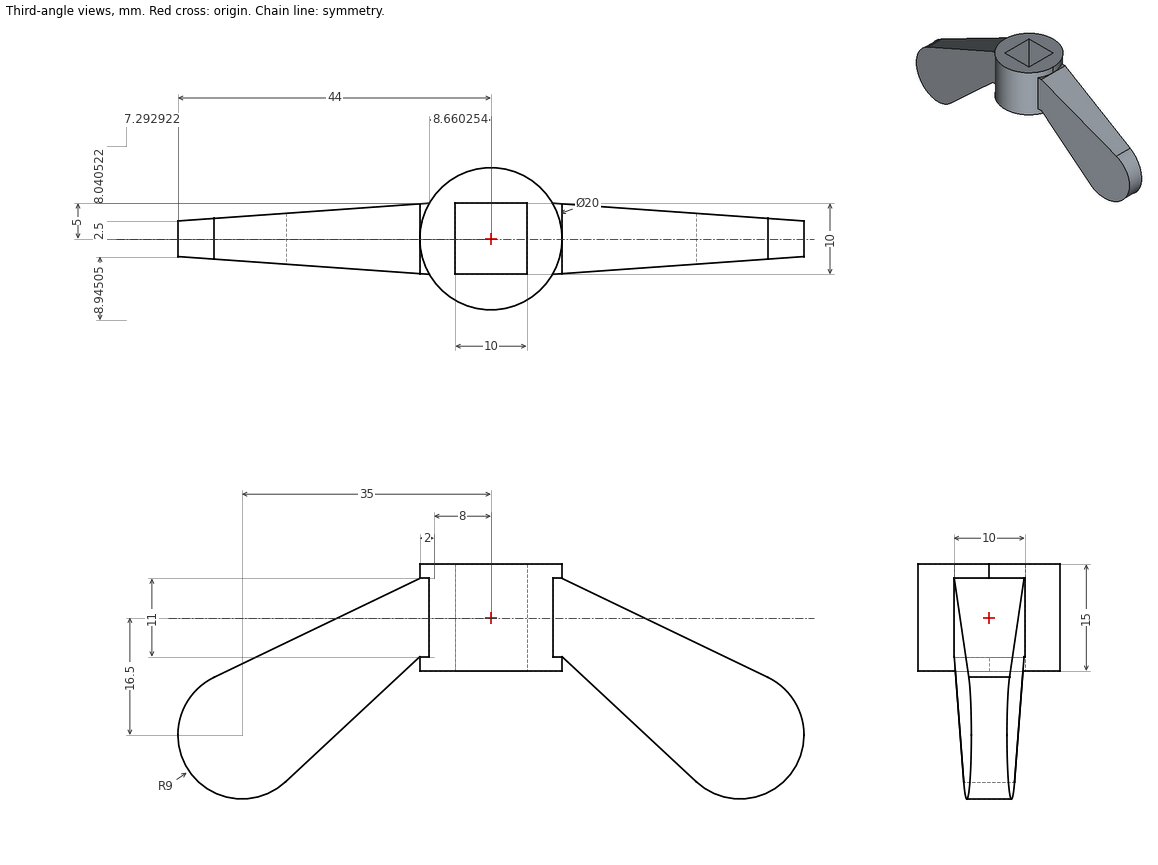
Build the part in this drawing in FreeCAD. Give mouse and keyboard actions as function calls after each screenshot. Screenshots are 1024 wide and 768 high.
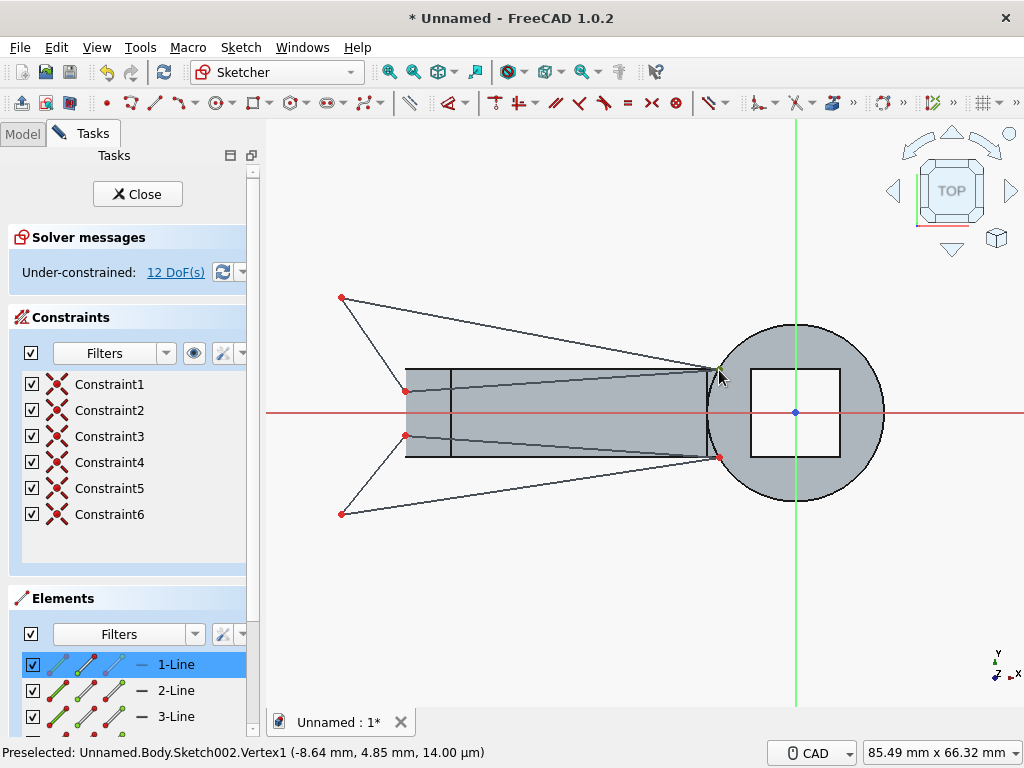
click(719, 458)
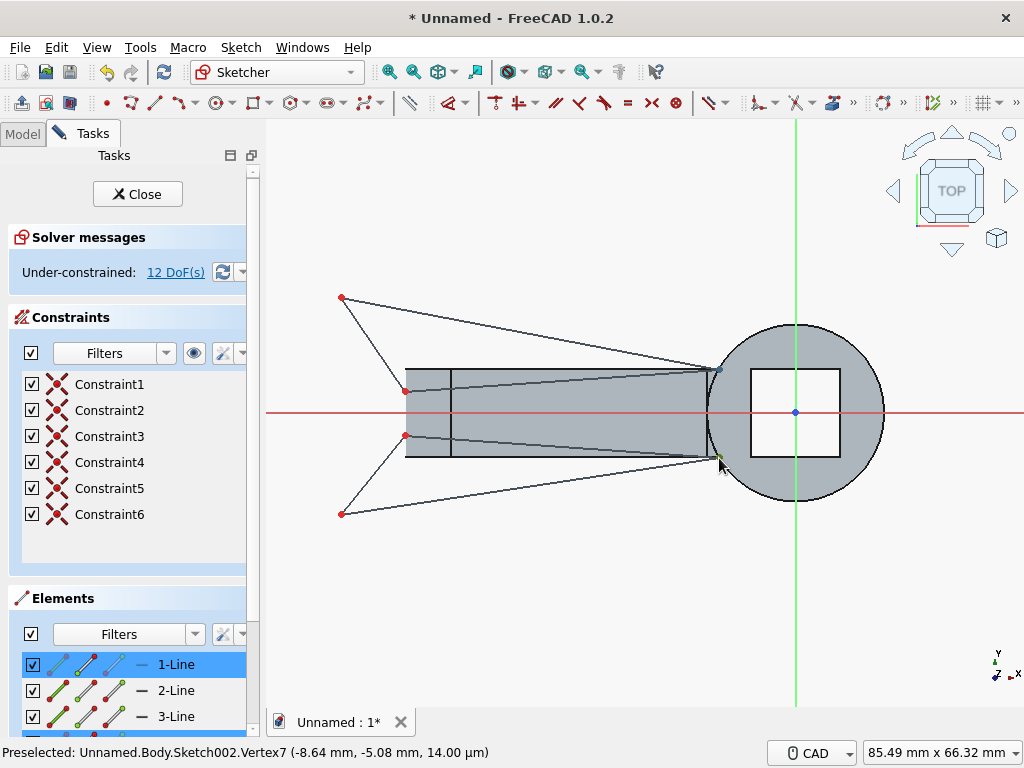
click(334, 413)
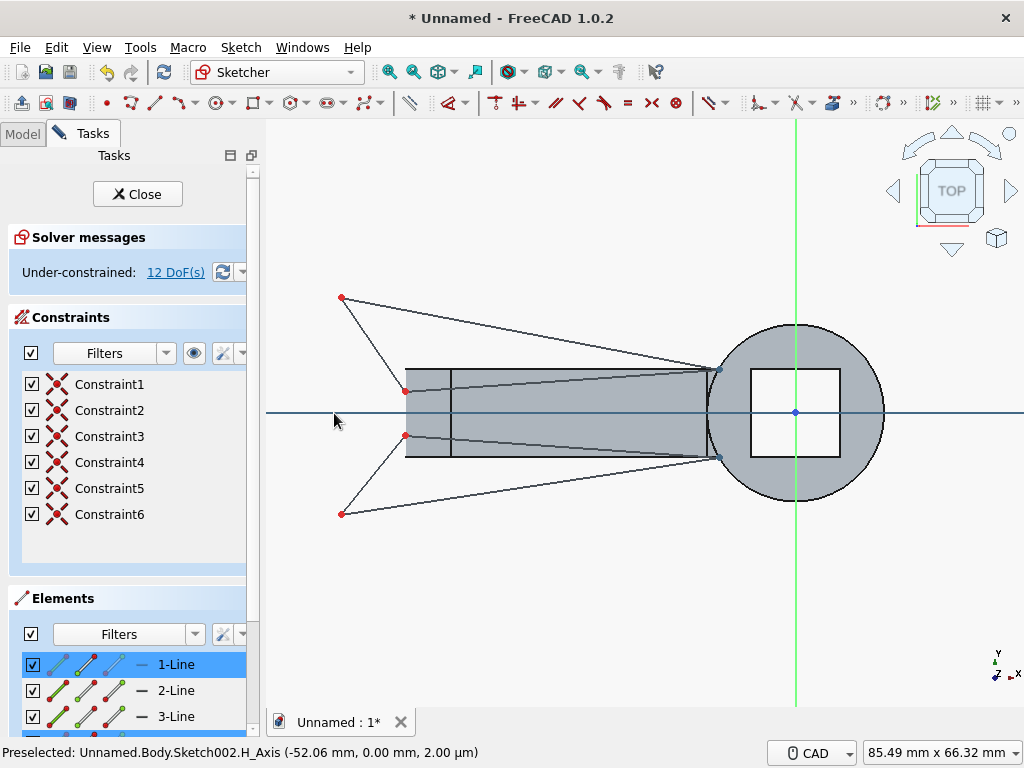
click(652, 104)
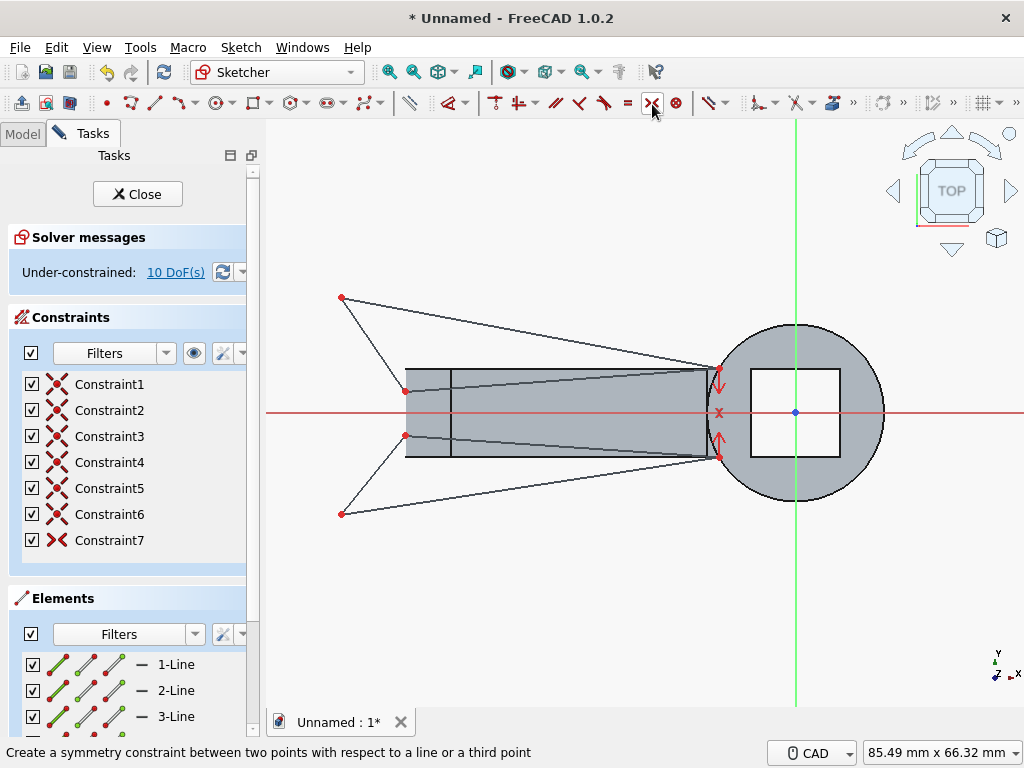
click(405, 392)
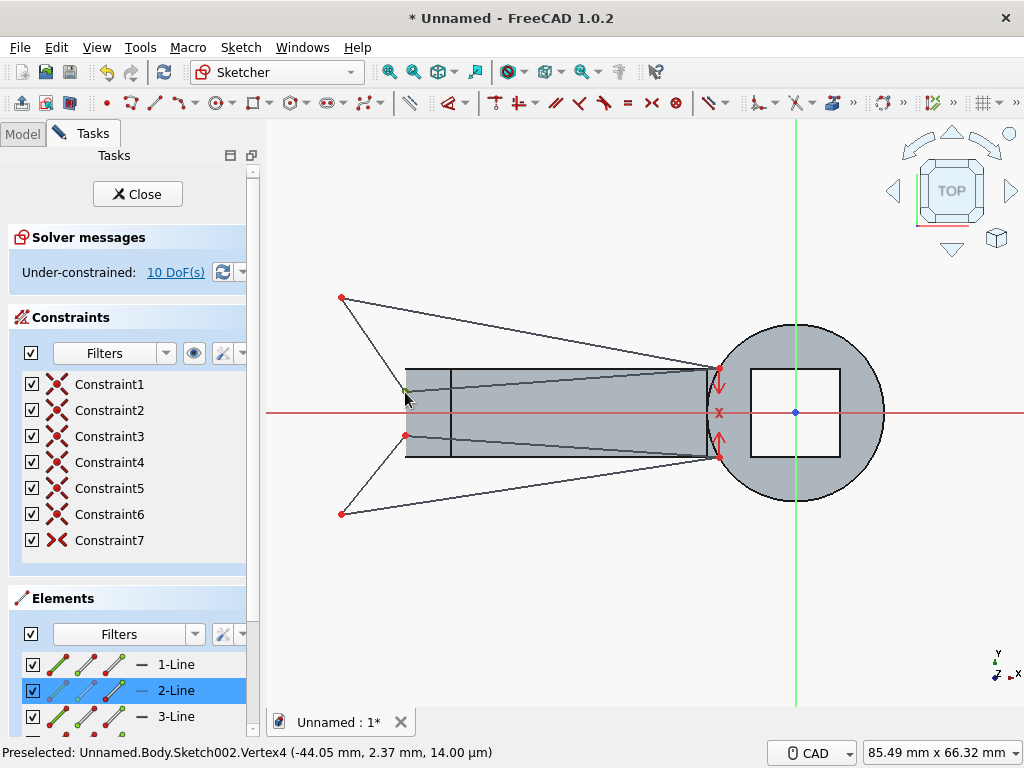
click(405, 436)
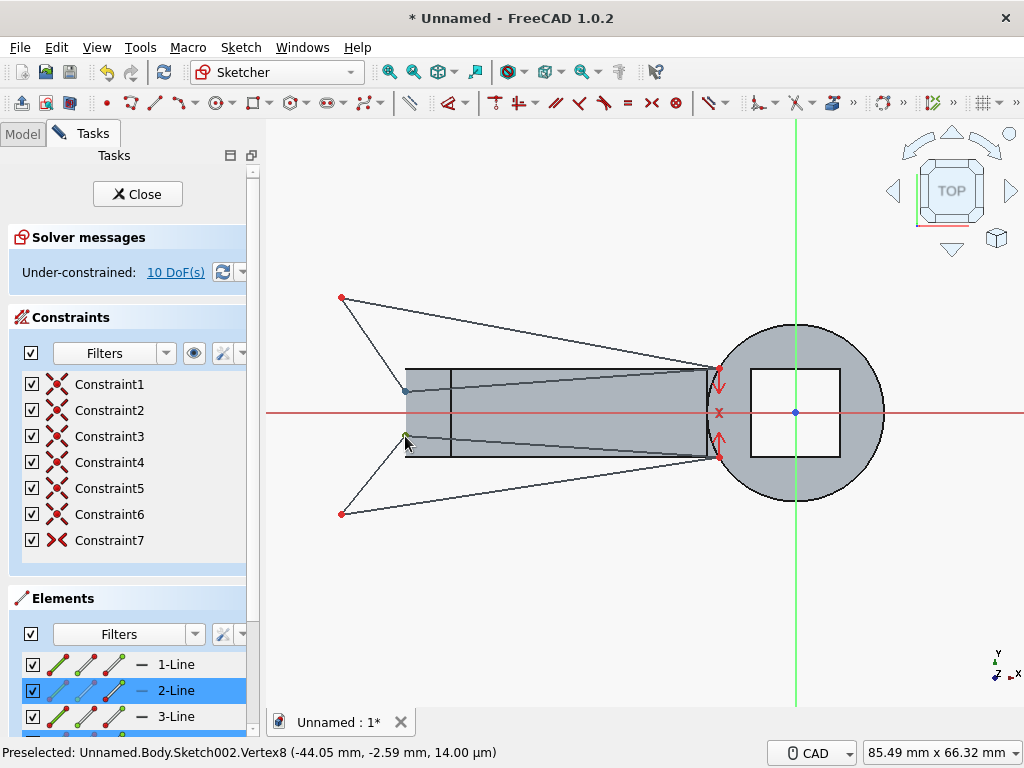
click(334, 413)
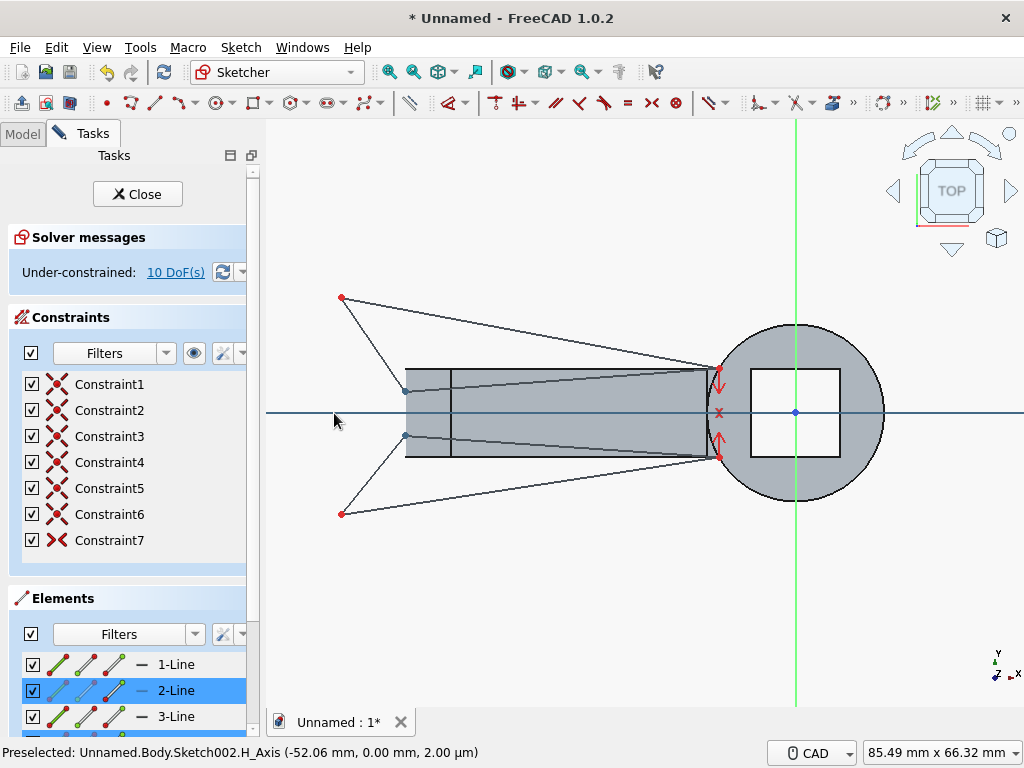
click(652, 104)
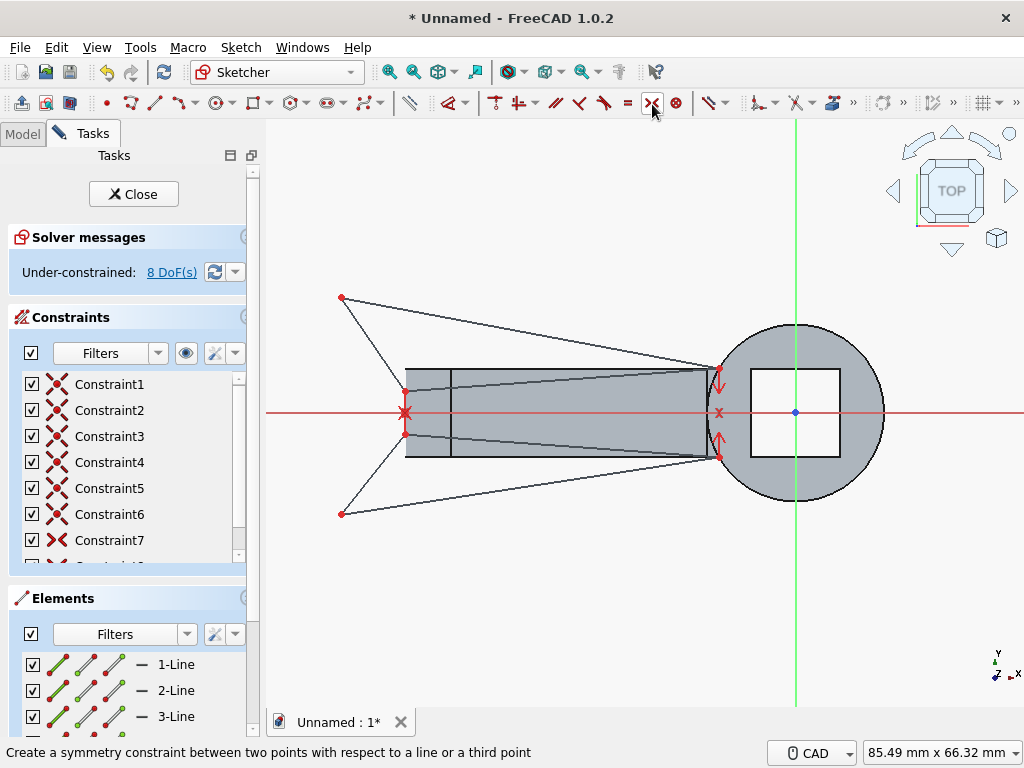
key(d)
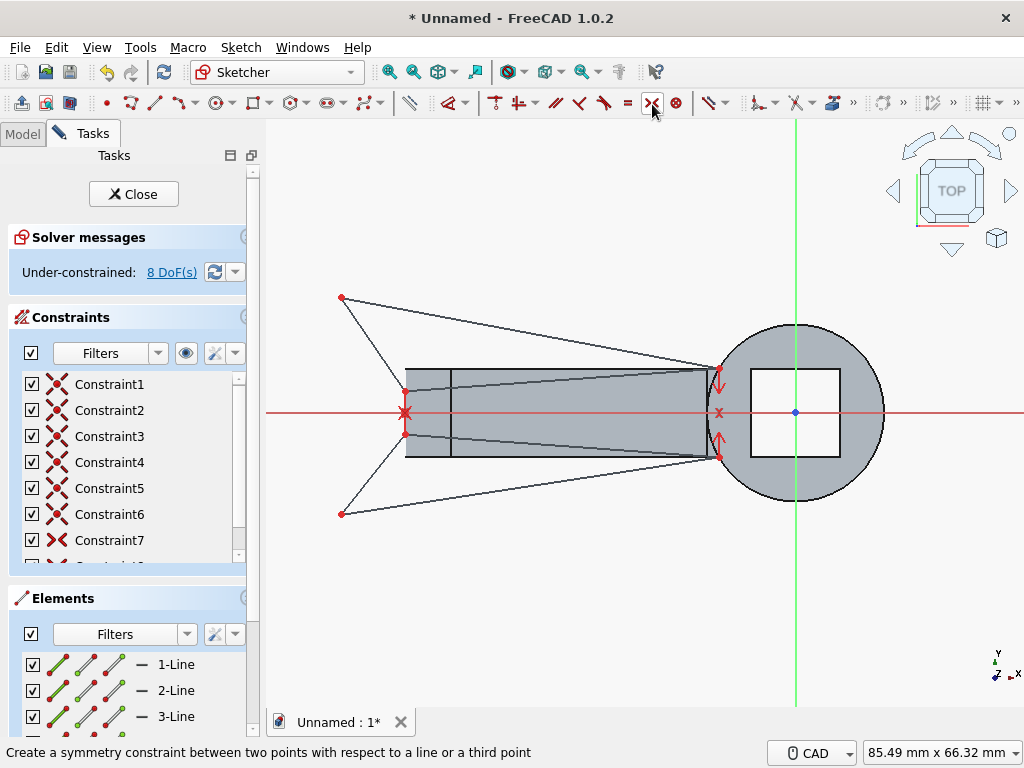
click(719, 369)
click(830, 391)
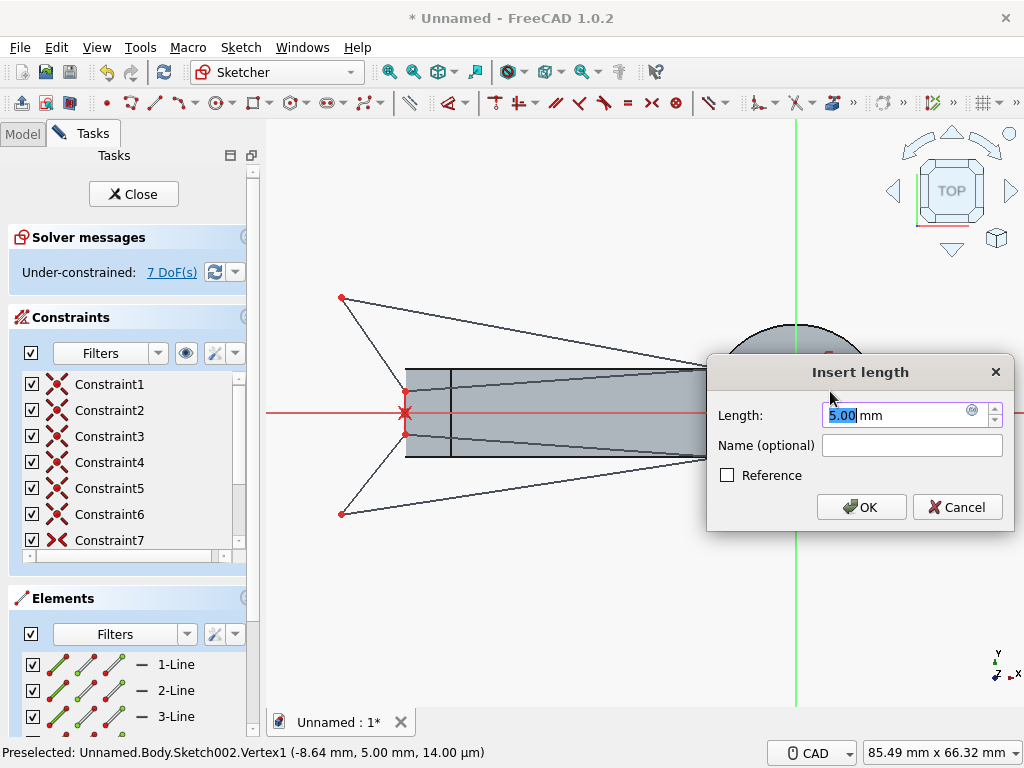
text(5)
key(Return)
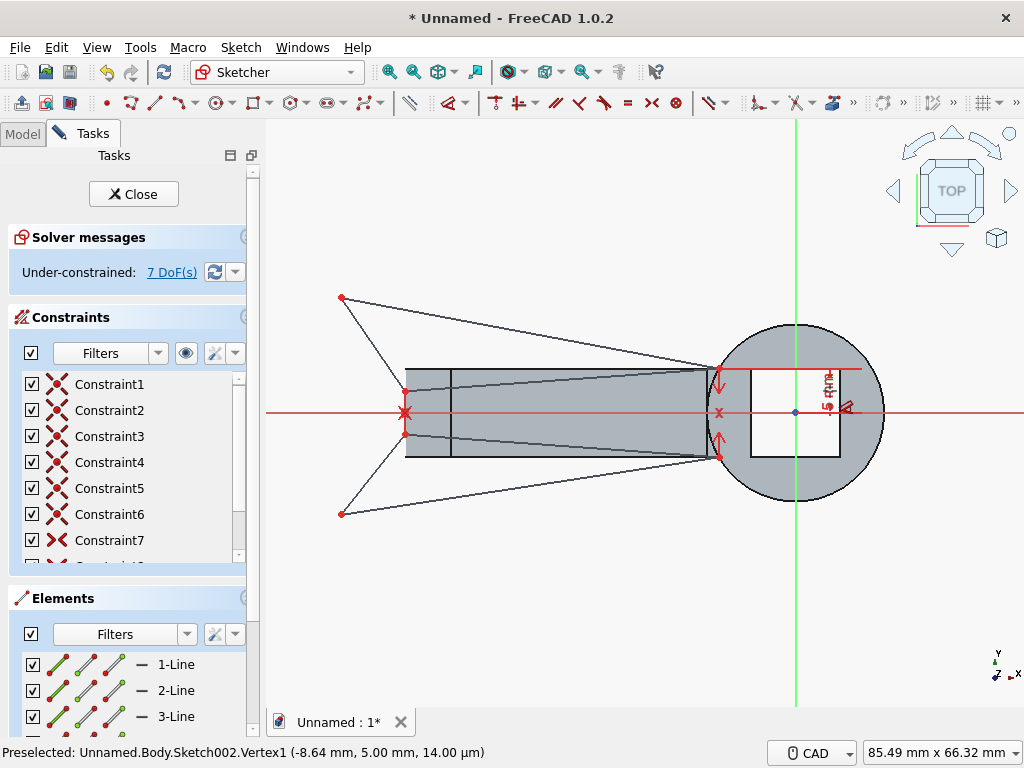
click(405, 391)
click(510, 357)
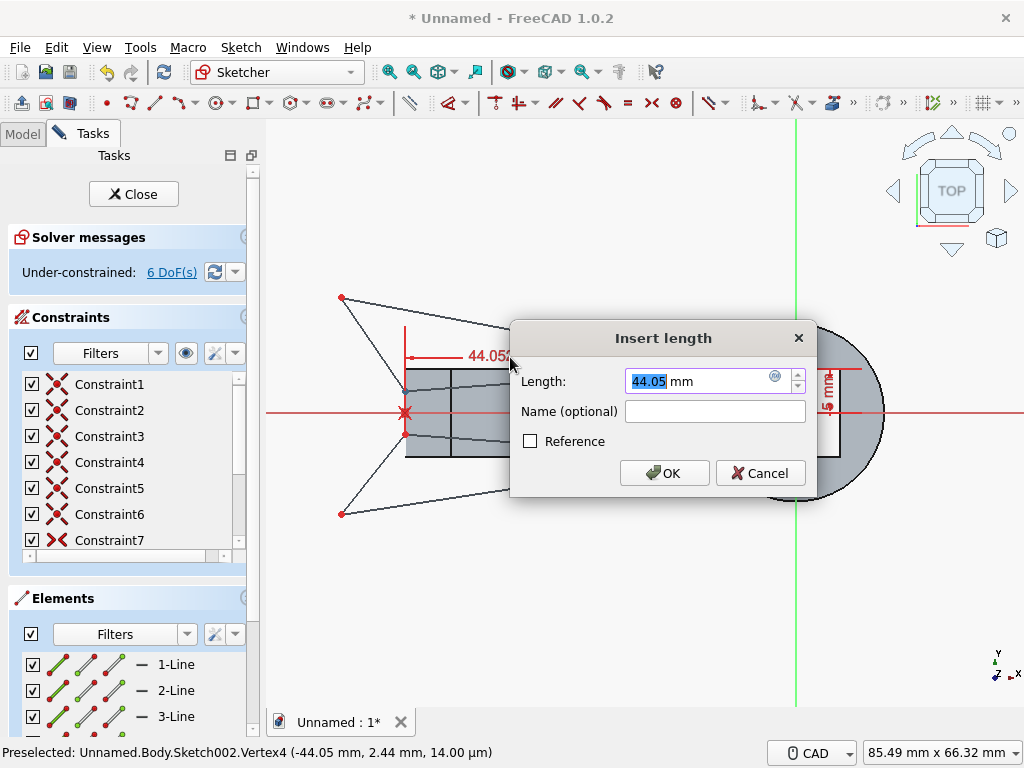
text(44)
key(Return)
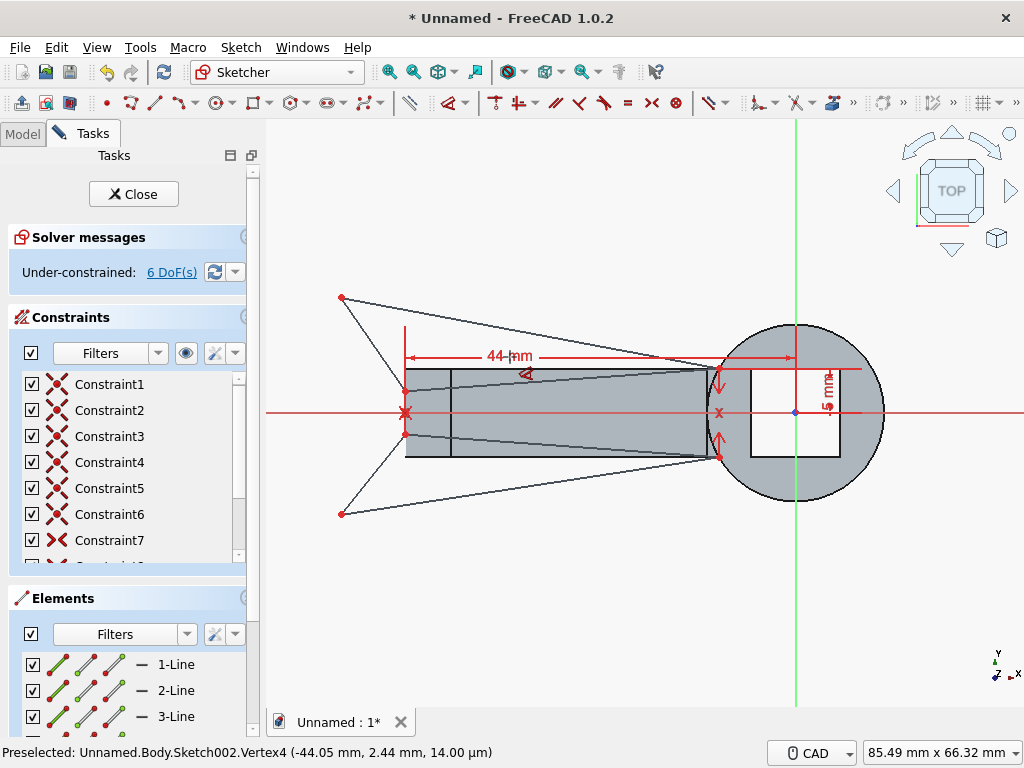
scroll(405, 391, up, 3)